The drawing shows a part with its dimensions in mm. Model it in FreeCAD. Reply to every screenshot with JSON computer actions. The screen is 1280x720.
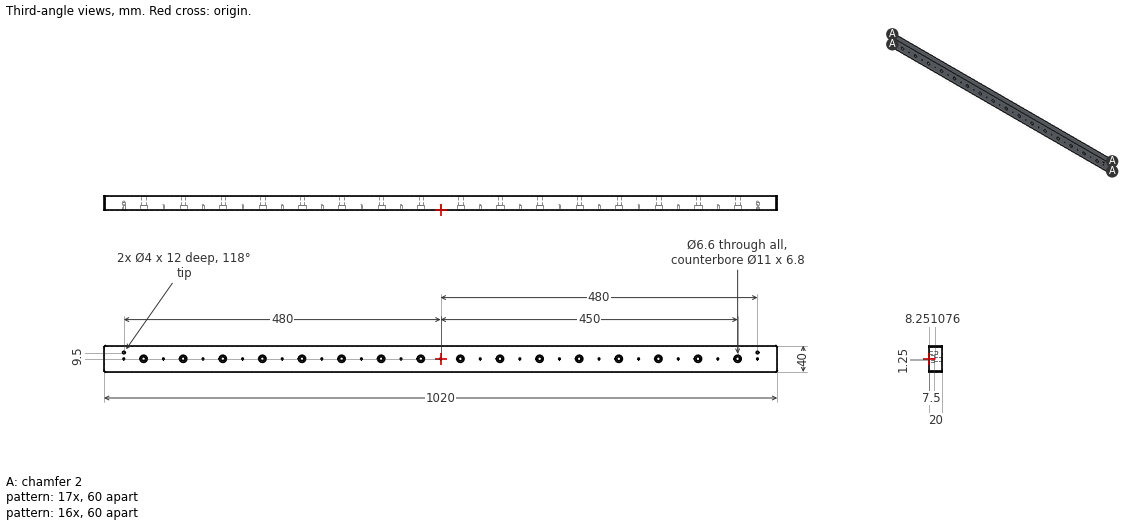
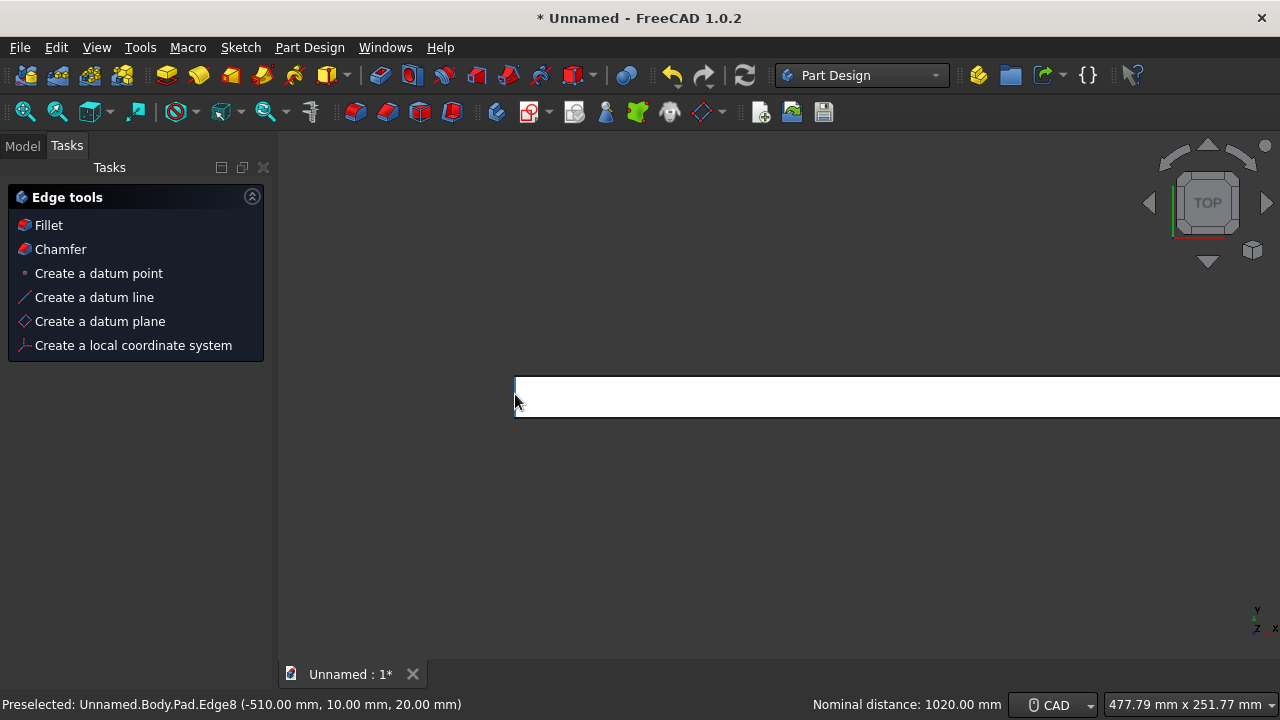
{"action": "left_click", "coordinate": [26, 112]}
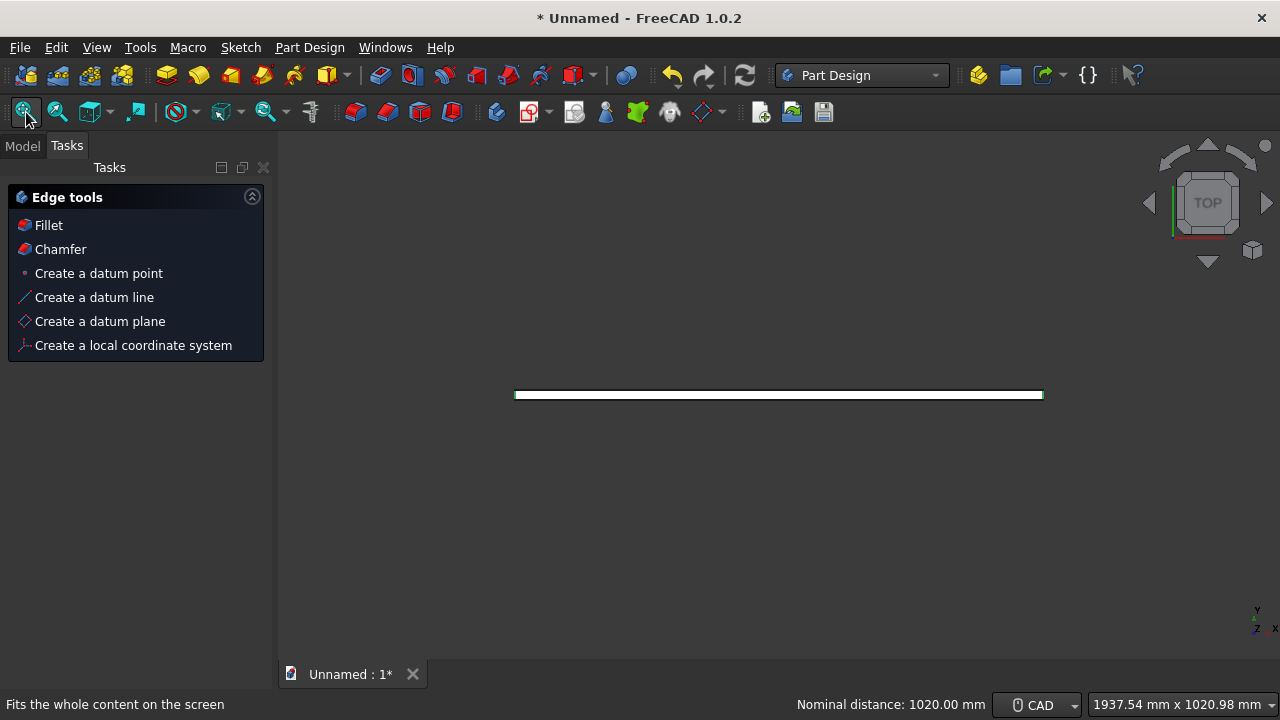
{"action": "key", "text": "1"}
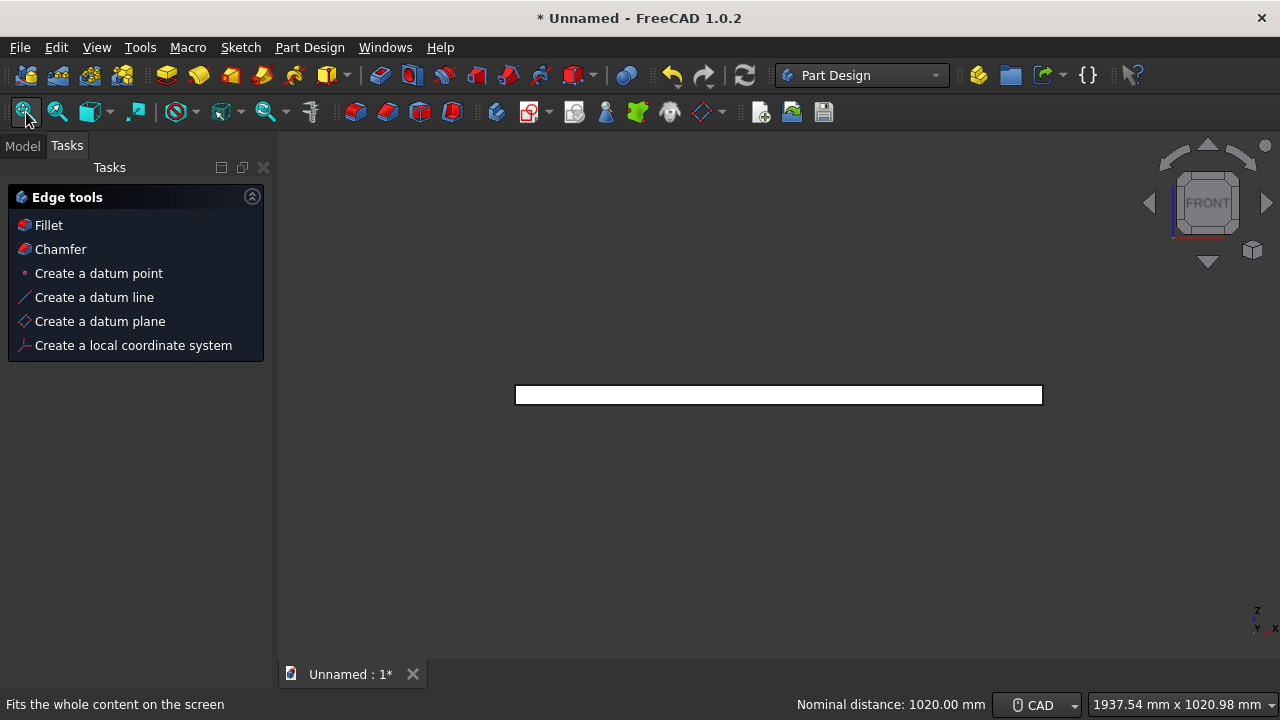
{"action": "scroll", "coordinate": [515, 404], "scroll_direction": "up", "scroll_amount": 7}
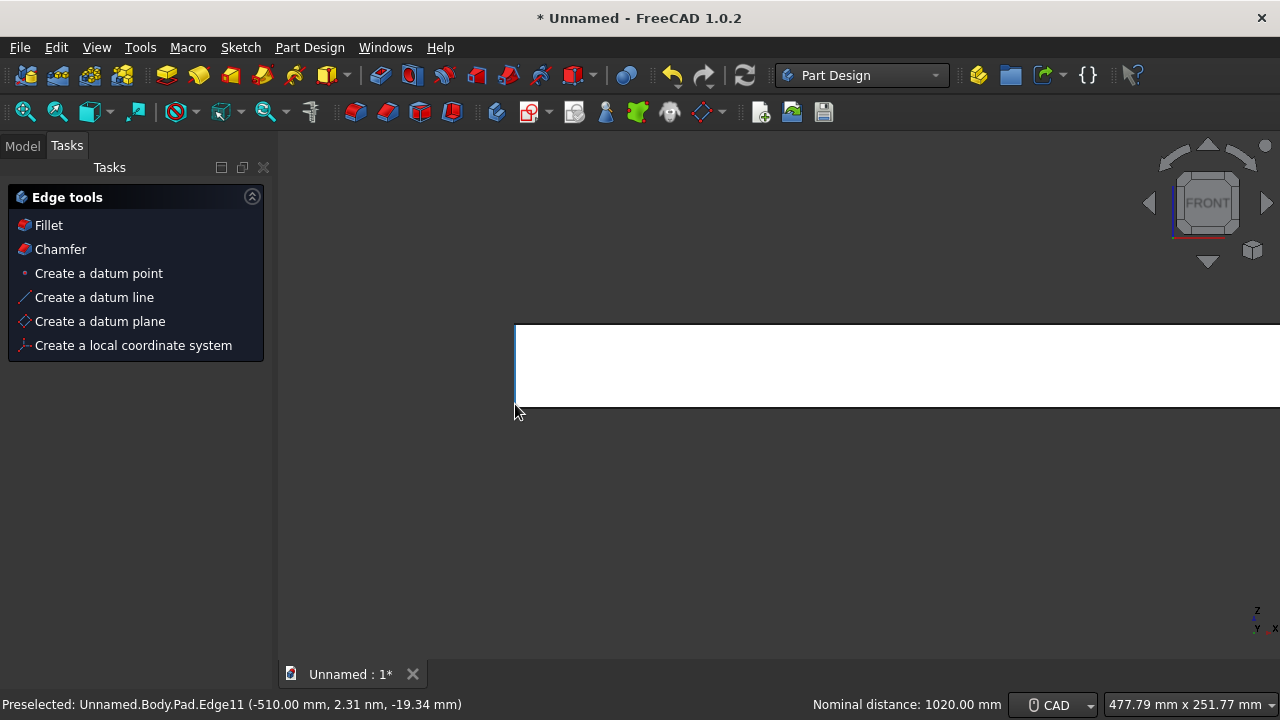
{"action": "key", "text": "v f"}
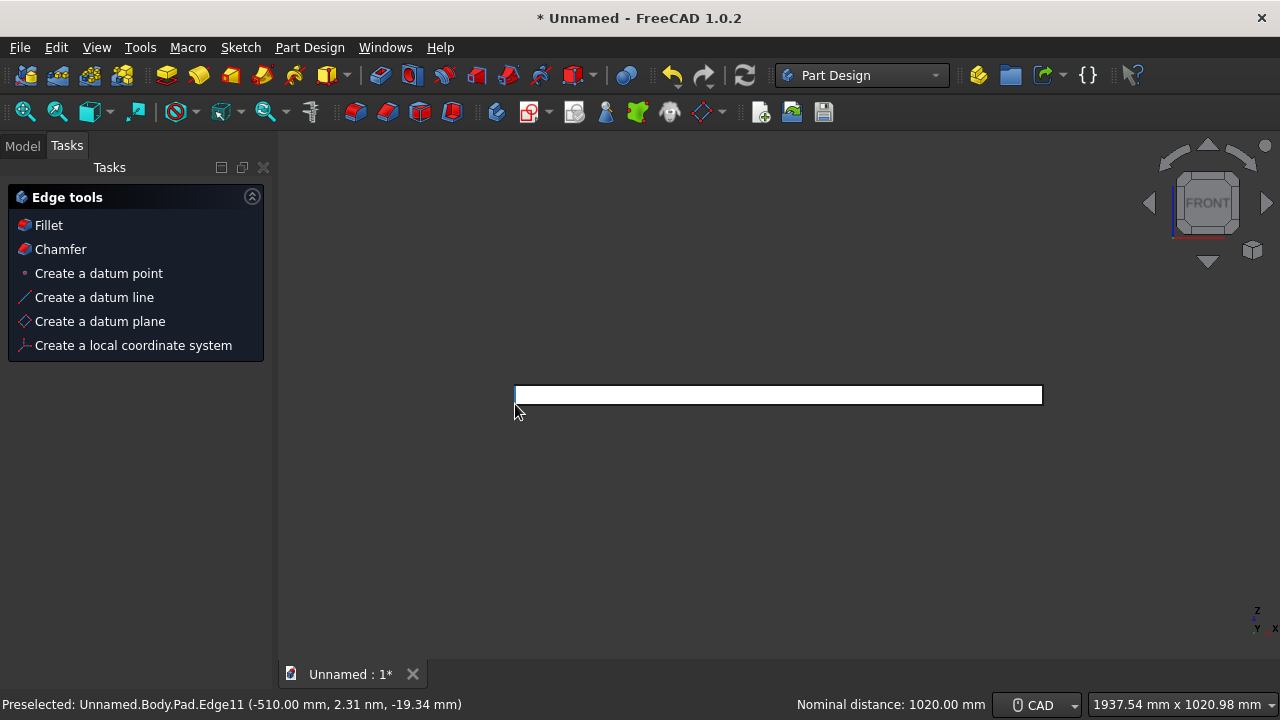
{"action": "key", "text": "3"}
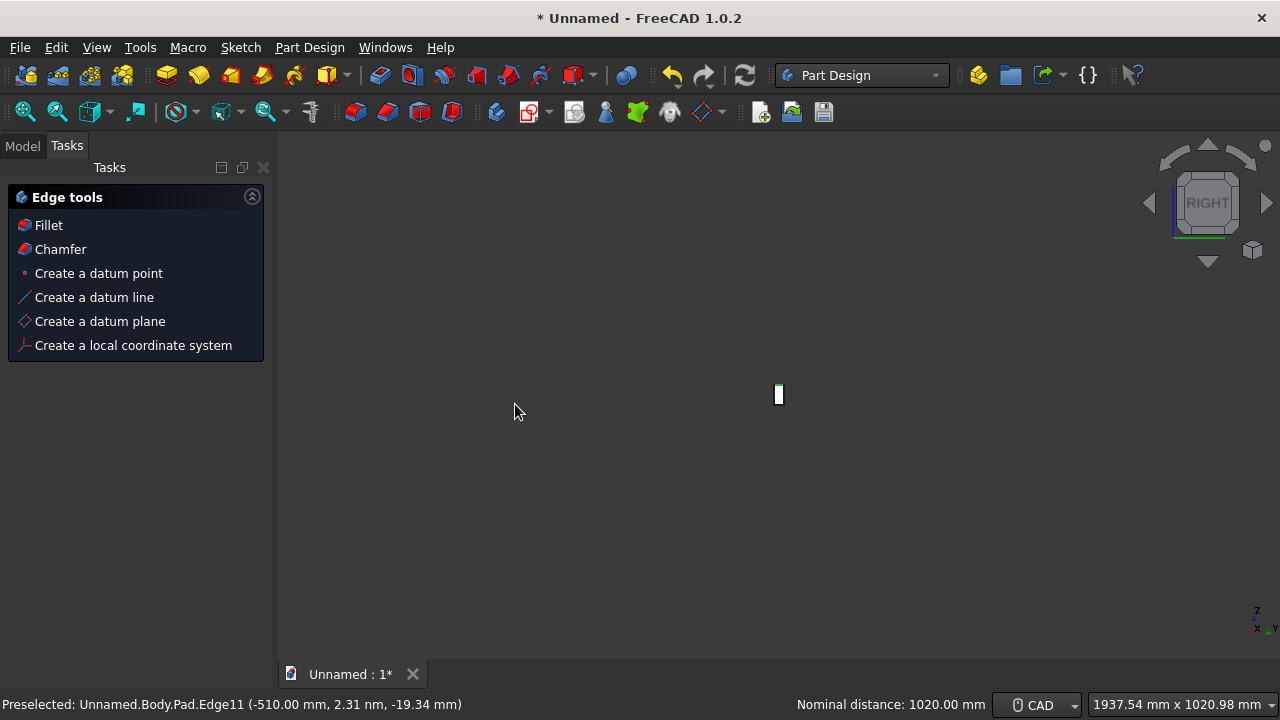
{"action": "key", "text": "v f"}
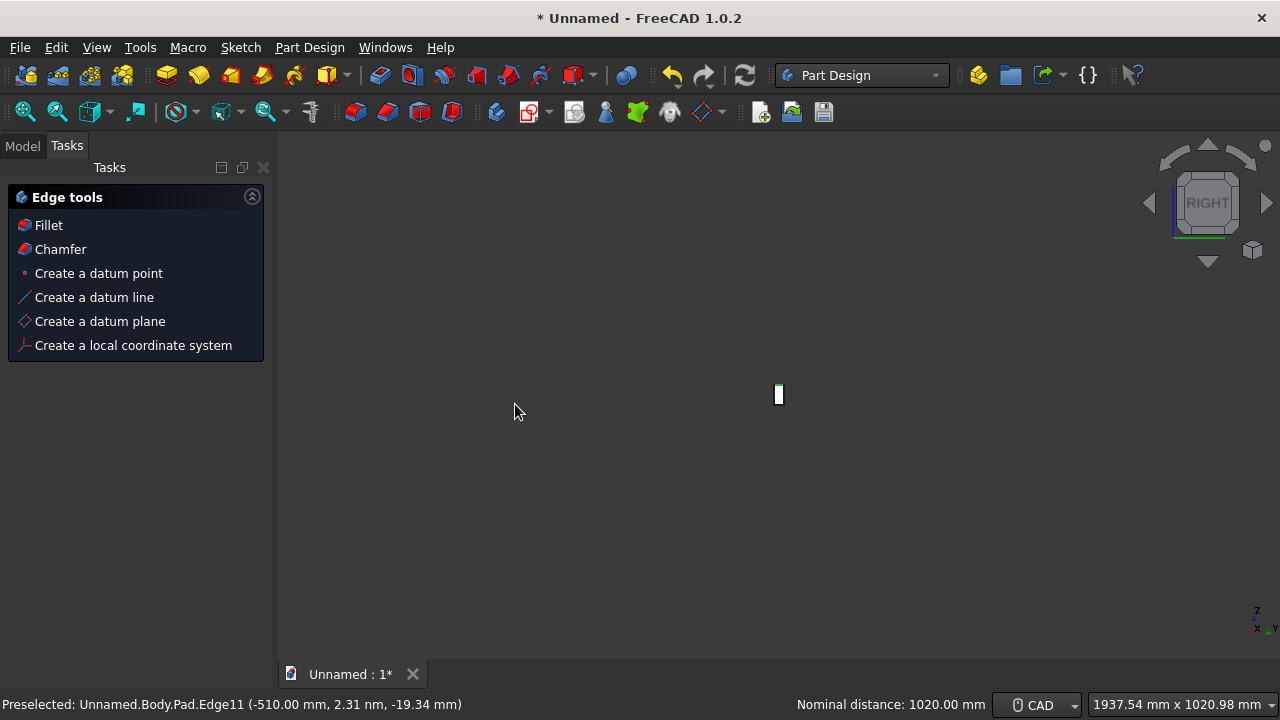
{"action": "scroll", "coordinate": [779, 404], "scroll_direction": "up", "scroll_amount": 7}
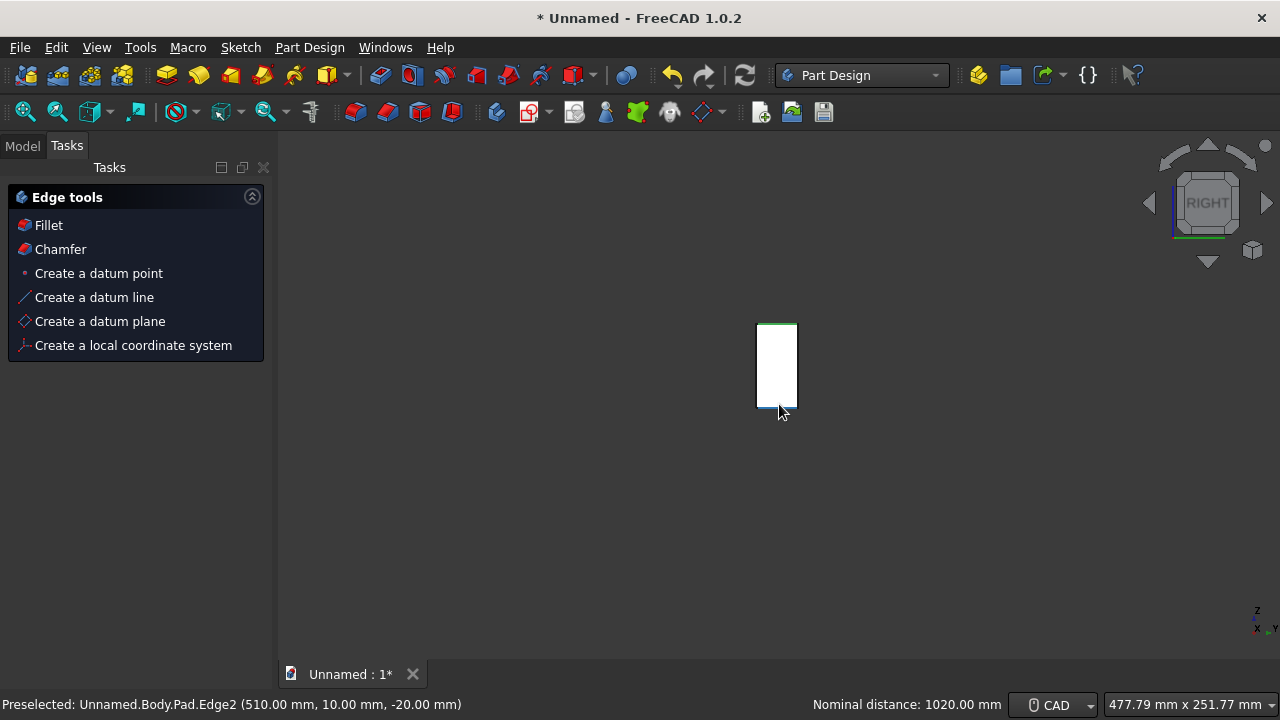
{"action": "left_click", "coordinate": [777, 407], "text": "ctrl"}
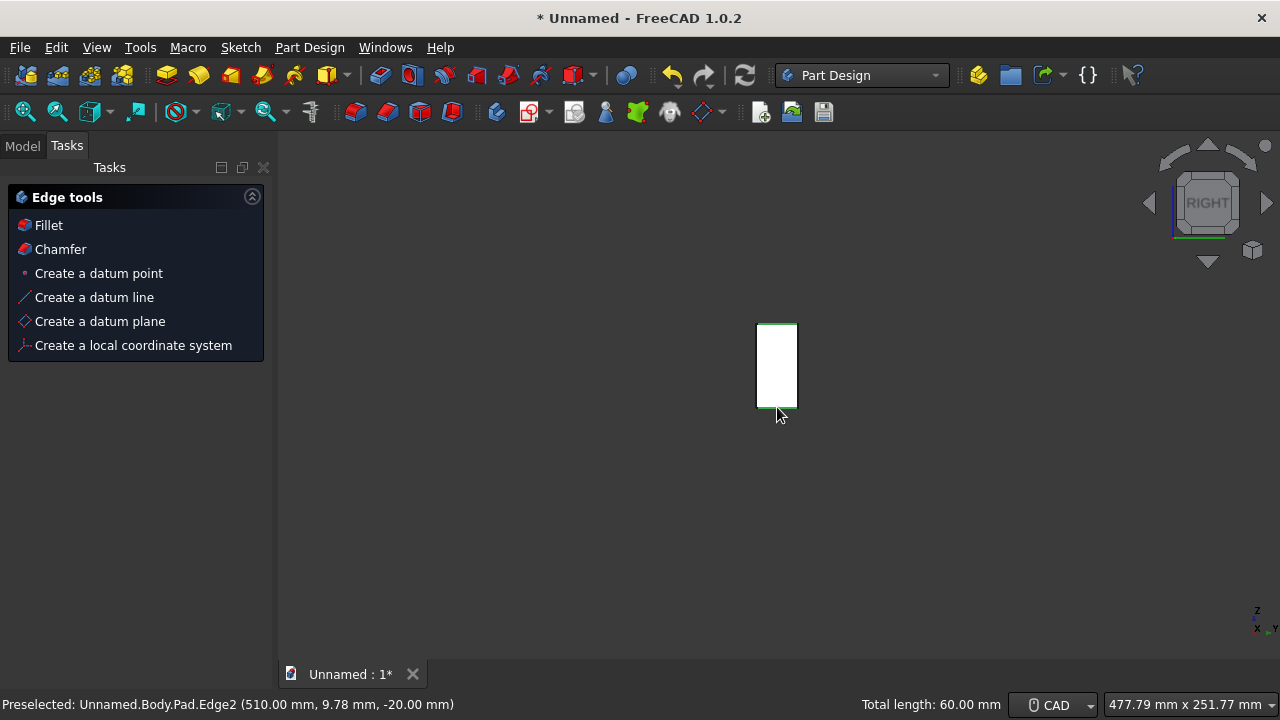
{"action": "key", "text": "v f"}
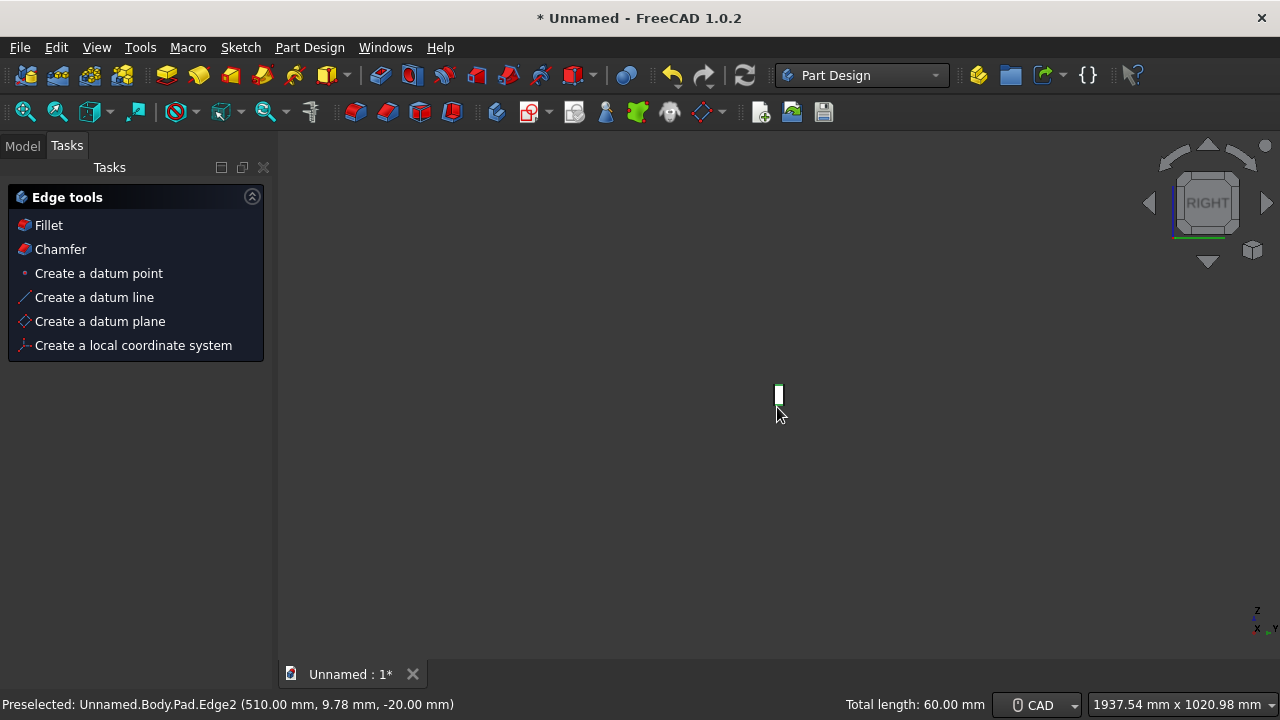
{"action": "key", "text": "5"}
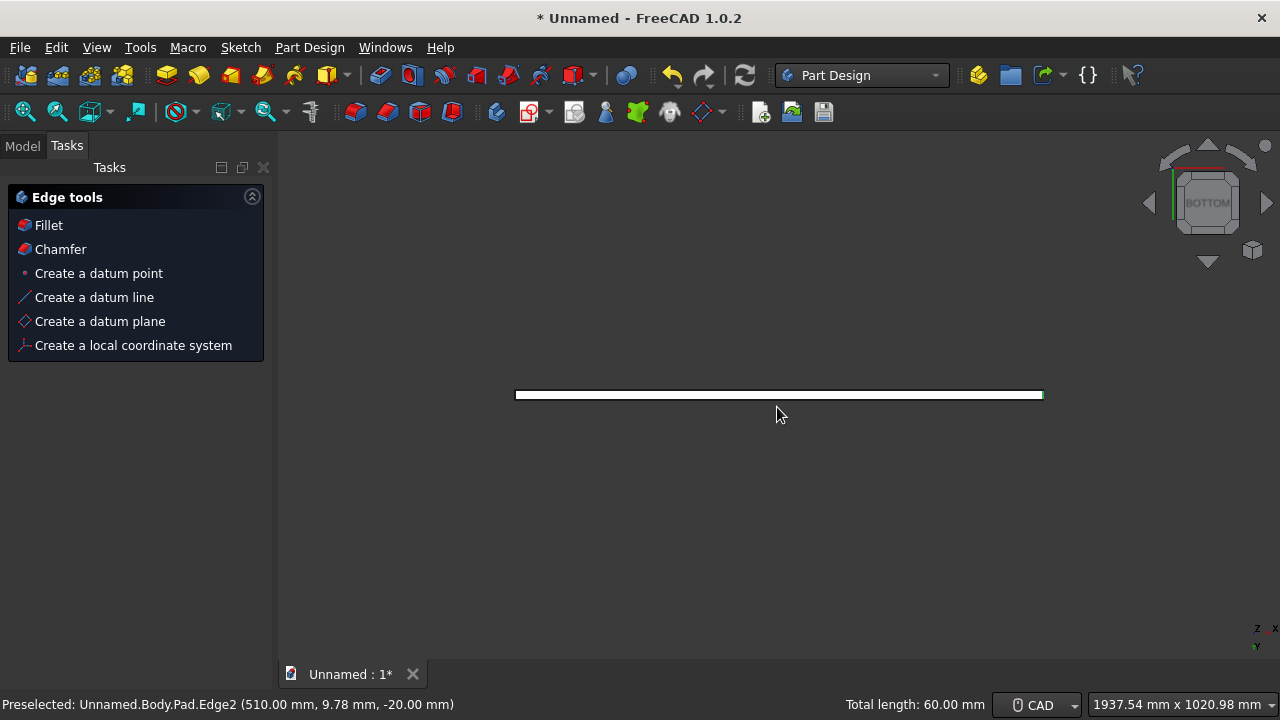
{"action": "left_click", "coordinate": [515, 395], "text": "ctrl"}